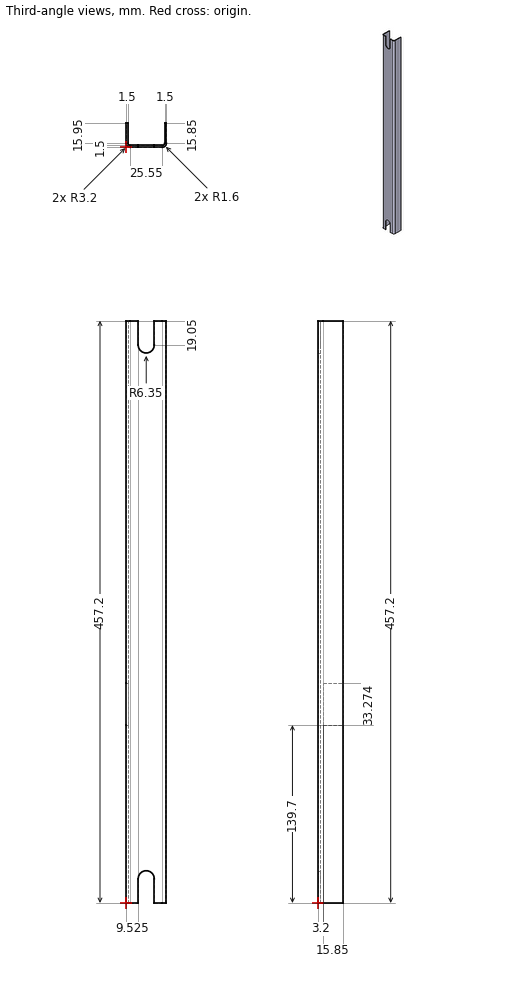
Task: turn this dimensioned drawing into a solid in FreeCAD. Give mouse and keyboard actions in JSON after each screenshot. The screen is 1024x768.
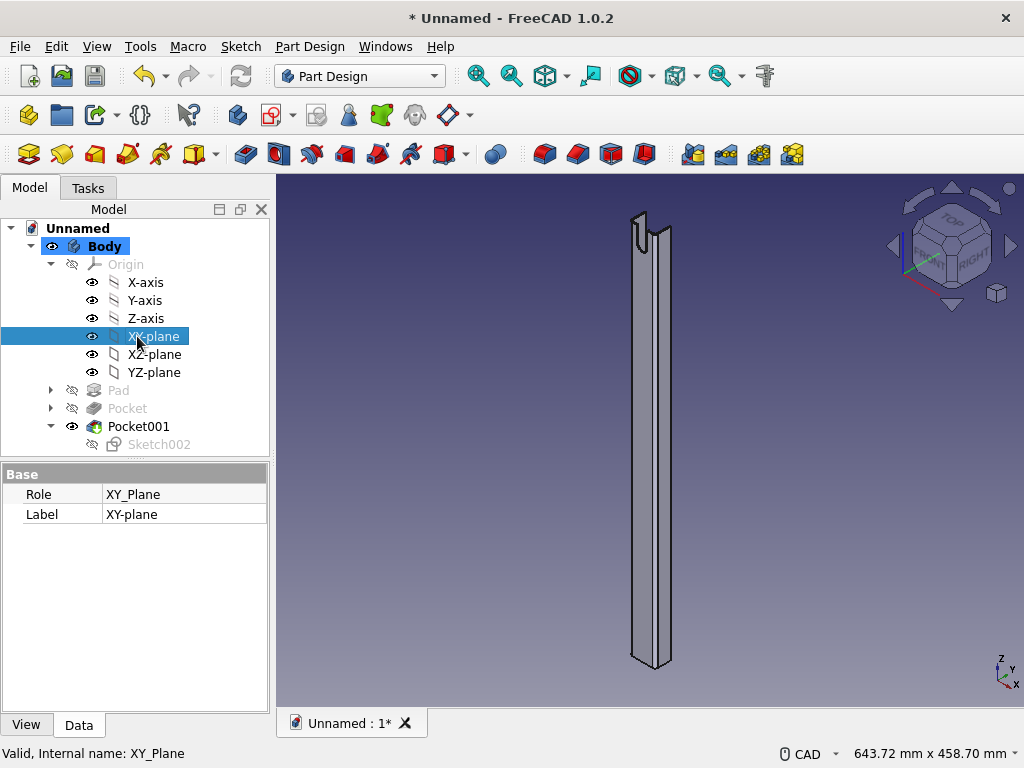
{"action": "left_click", "coordinate": [448, 116]}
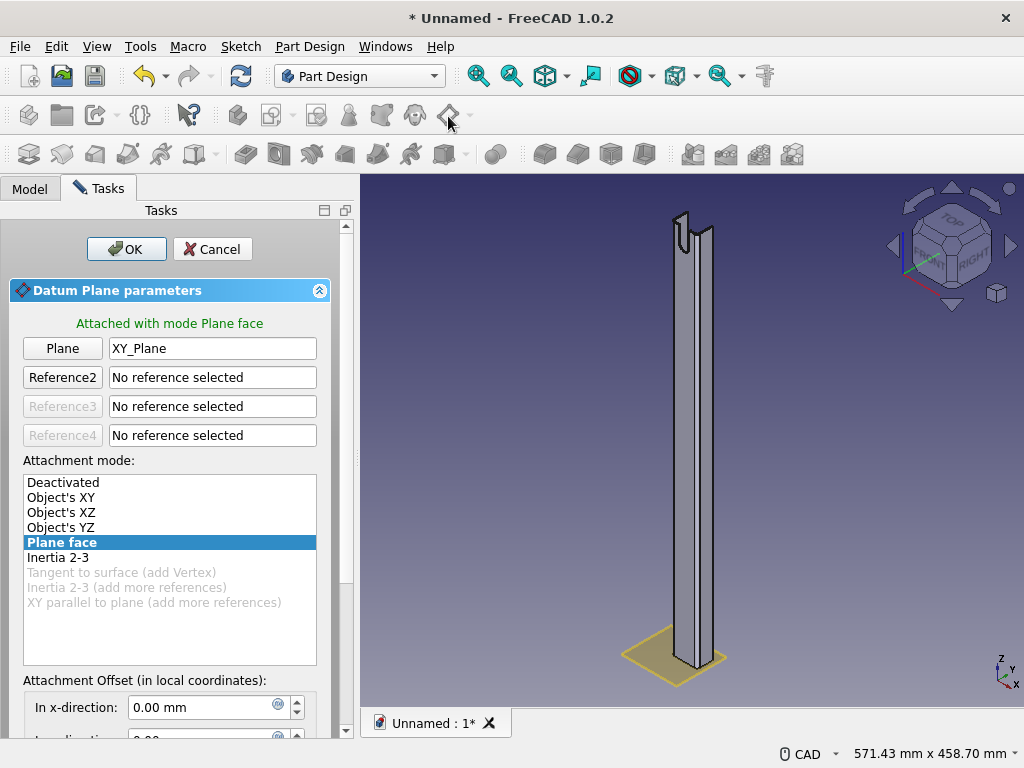
{"action": "scroll", "coordinate": [346, 479], "scroll_direction": "down", "scroll_amount": 2}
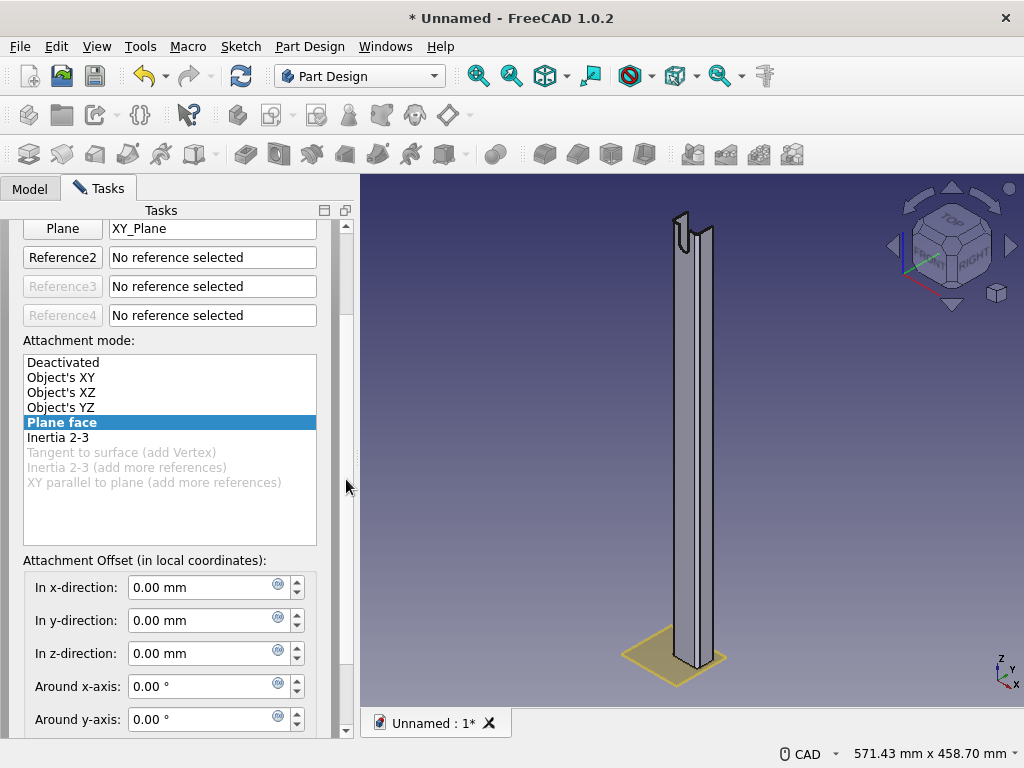
{"action": "triple_click", "coordinate": [210, 654]}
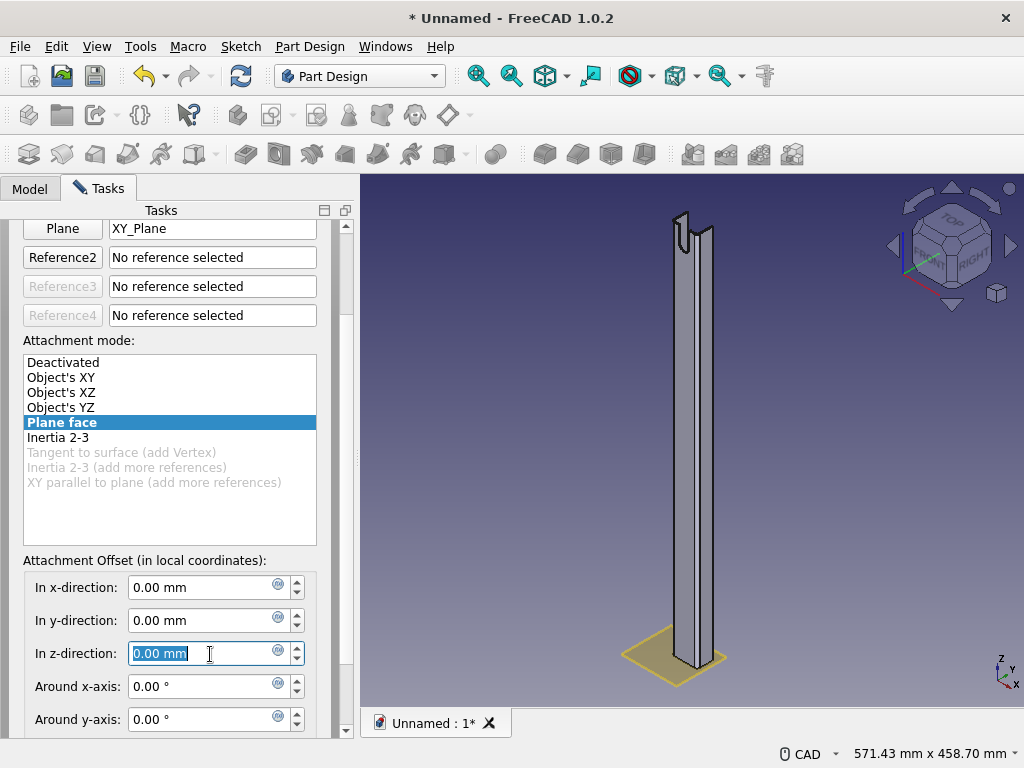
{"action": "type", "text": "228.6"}
{"action": "key", "text": "Tab"}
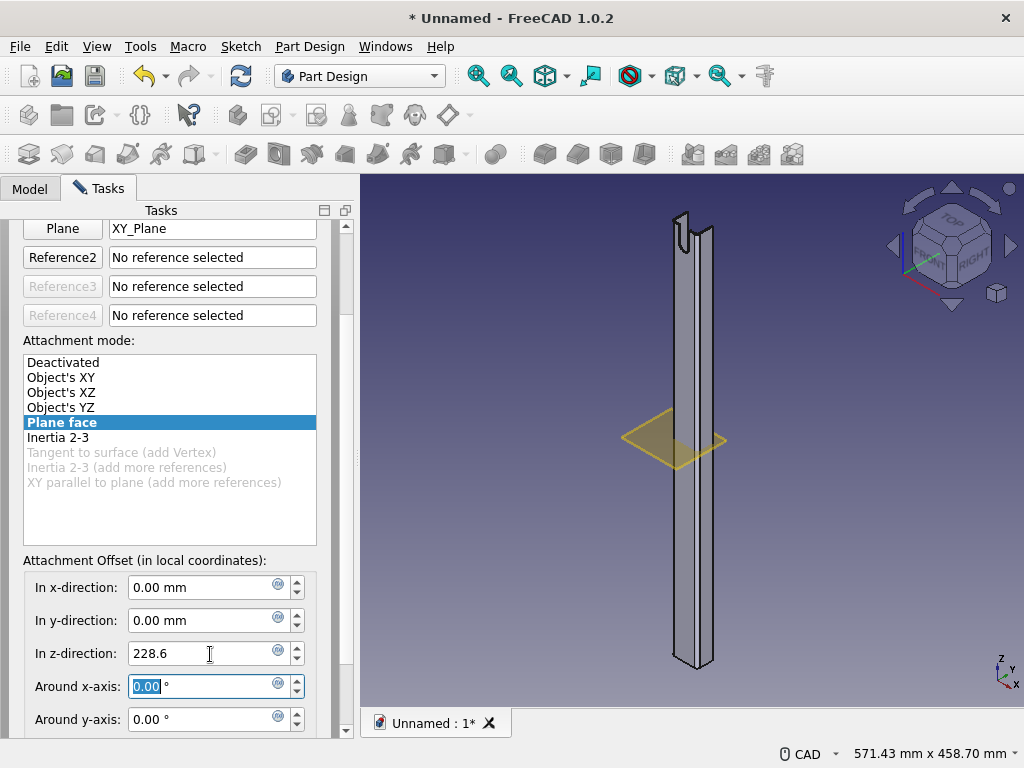
{"action": "scroll", "coordinate": [346, 479], "scroll_direction": "up", "scroll_amount": 3}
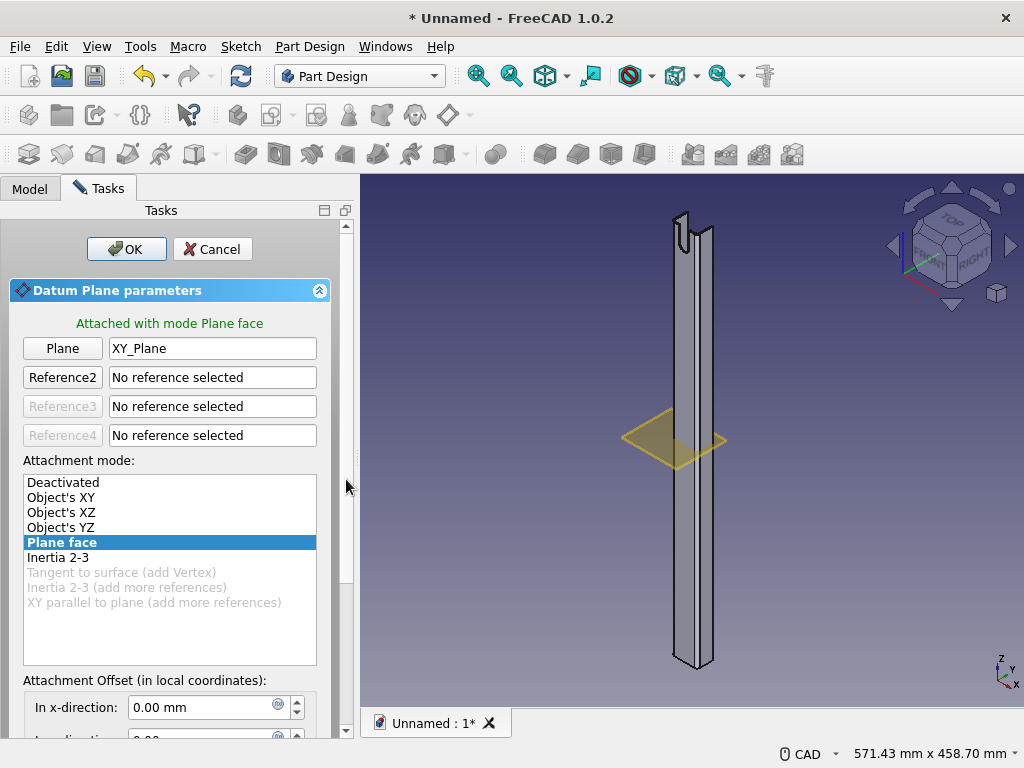
{"action": "left_click", "coordinate": [127, 249]}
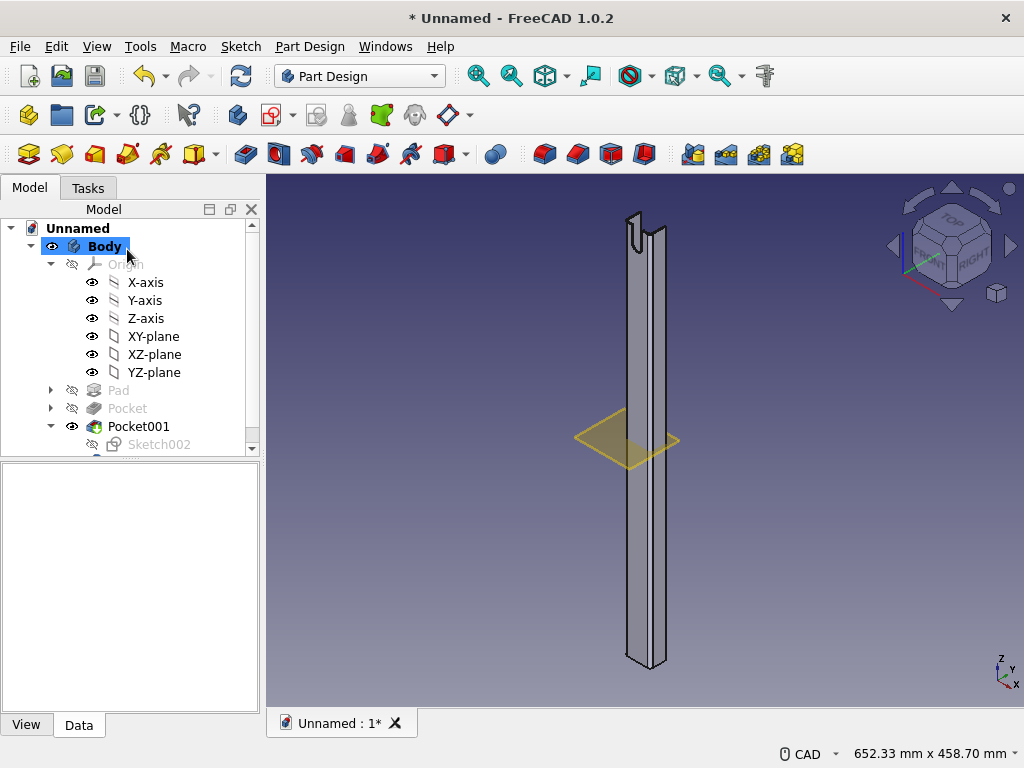
{"action": "left_click", "coordinate": [117, 426]}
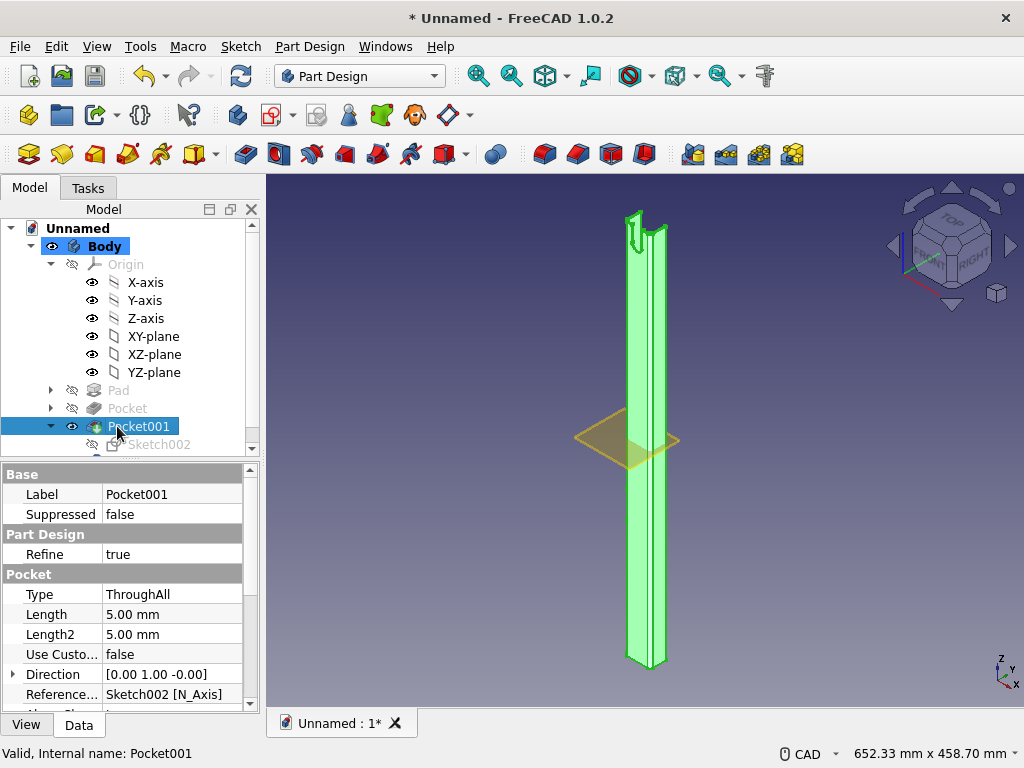
{"action": "left_click", "coordinate": [693, 154]}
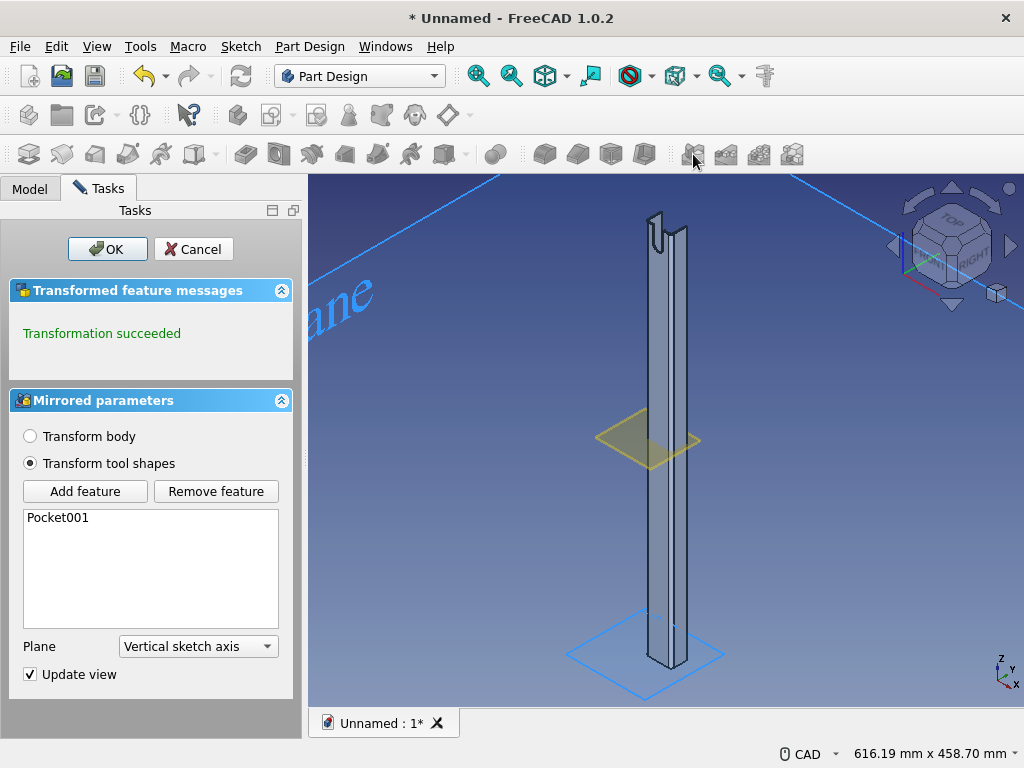
{"action": "left_click", "coordinate": [199, 646]}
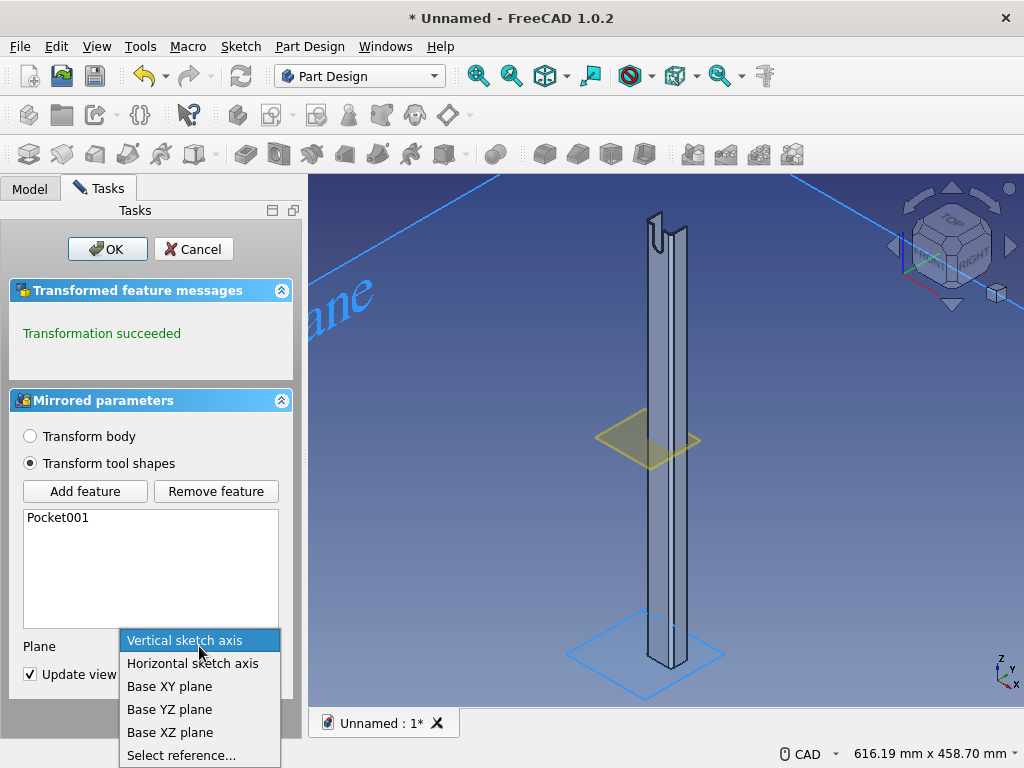
{"action": "left_click", "coordinate": [198, 756]}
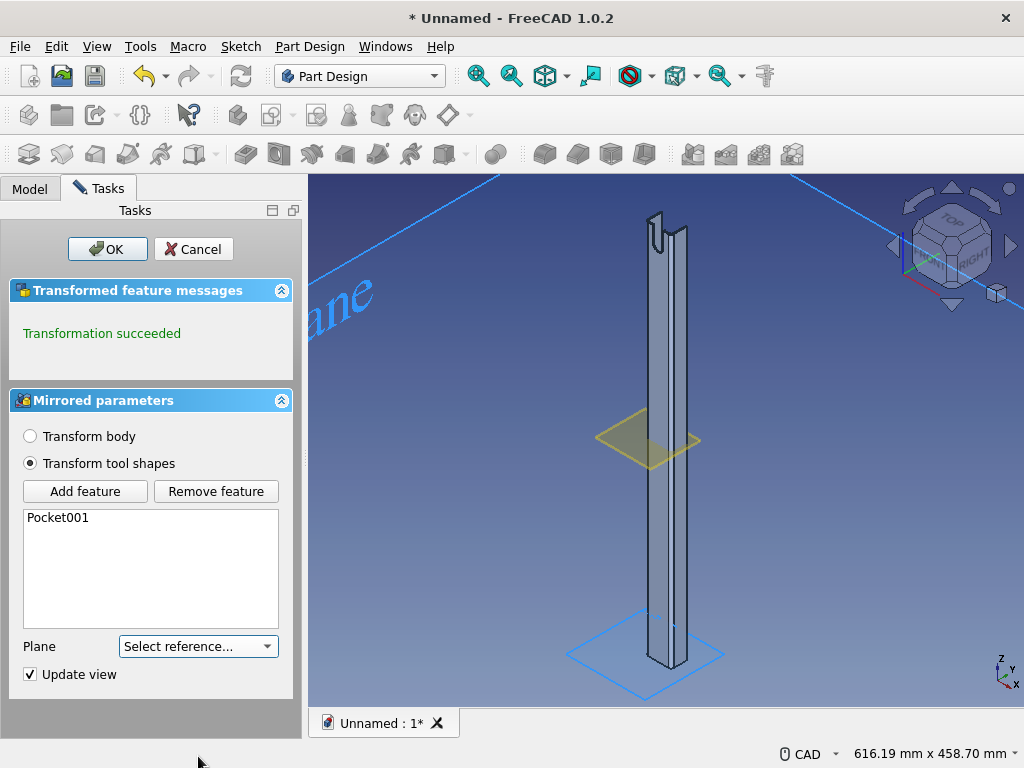
{"action": "left_click", "coordinate": [30, 188]}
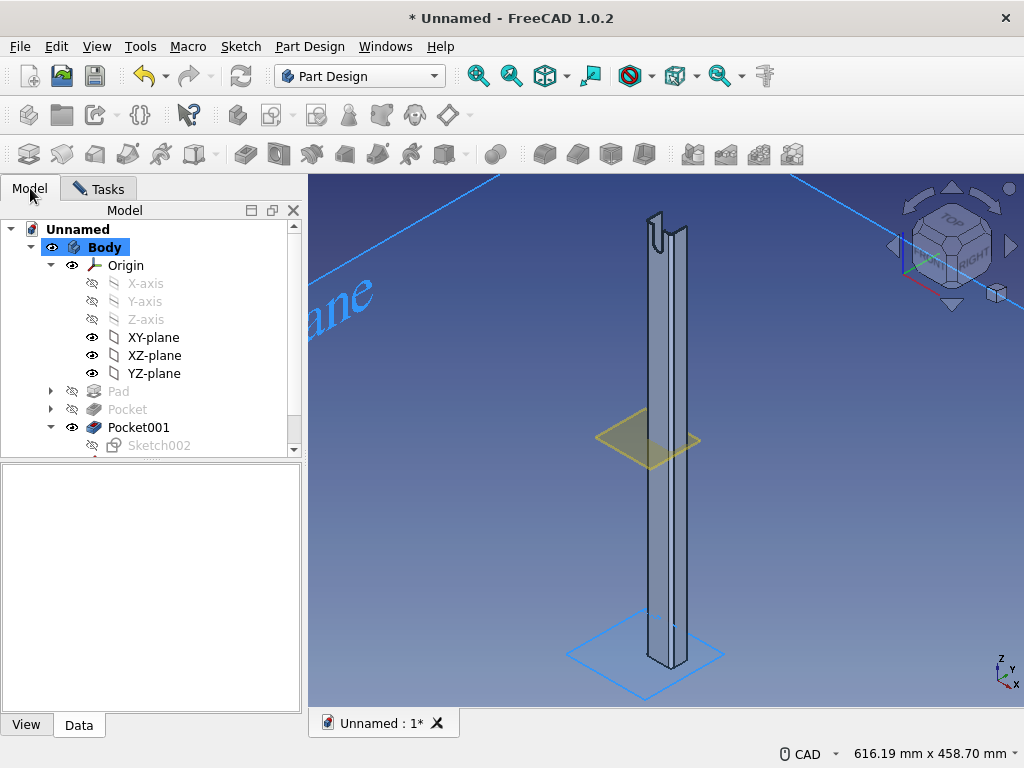
{"action": "scroll", "coordinate": [101, 333], "scroll_direction": "down", "scroll_amount": 3}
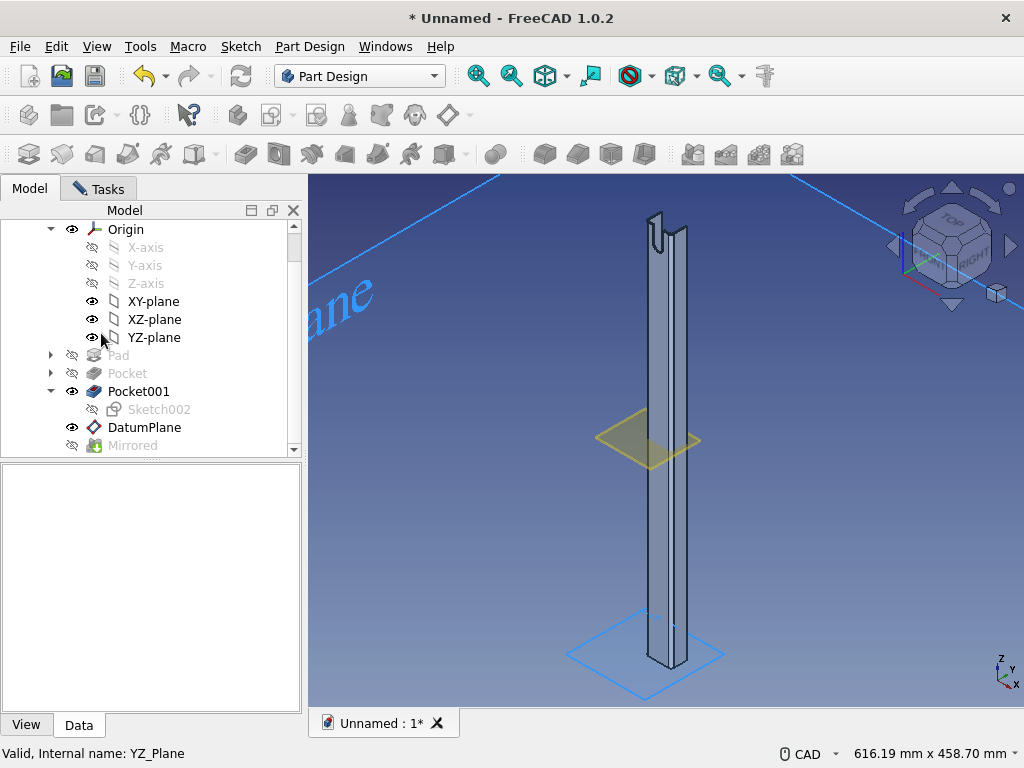
{"action": "left_click", "coordinate": [117, 427]}